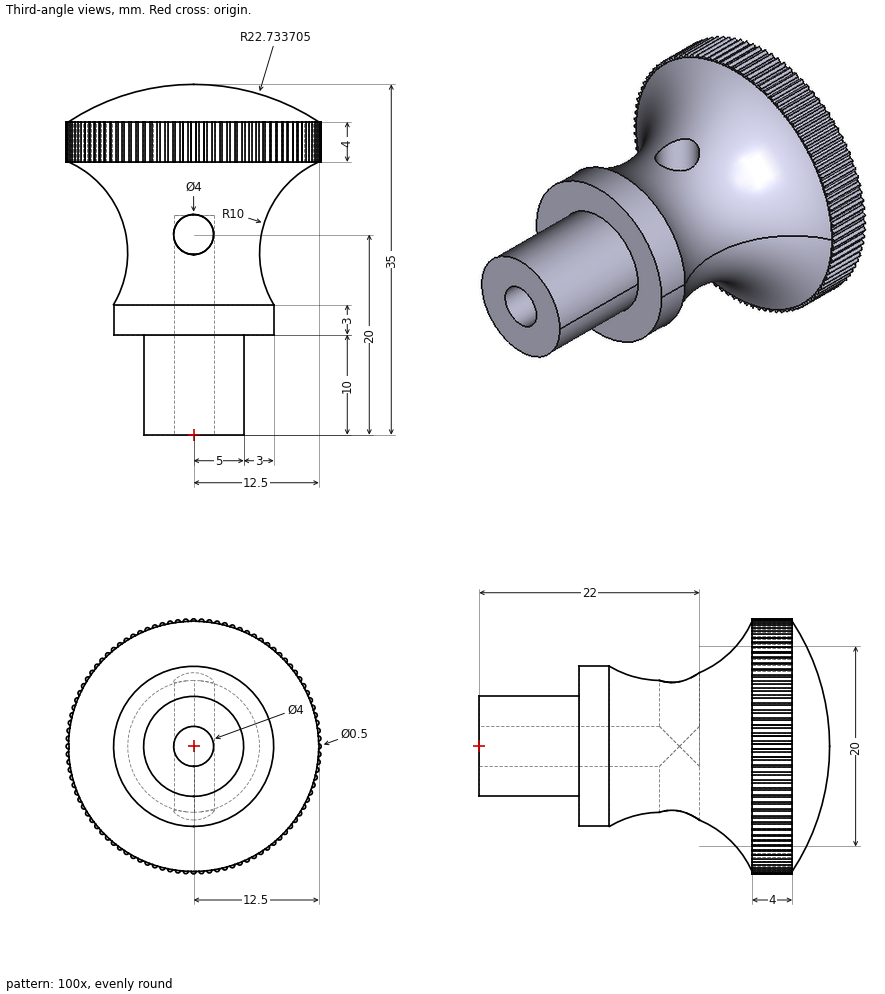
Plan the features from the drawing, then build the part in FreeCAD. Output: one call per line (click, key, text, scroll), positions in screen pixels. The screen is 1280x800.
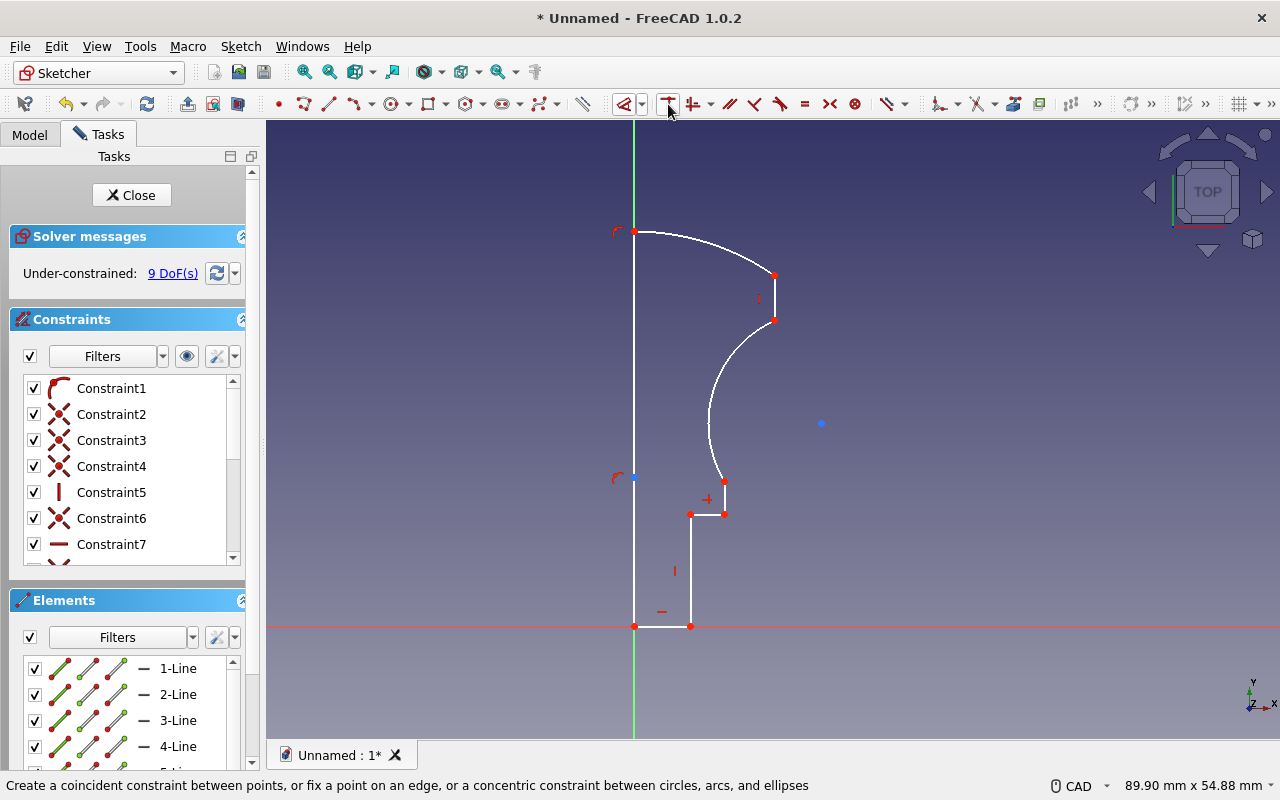
click(624, 104)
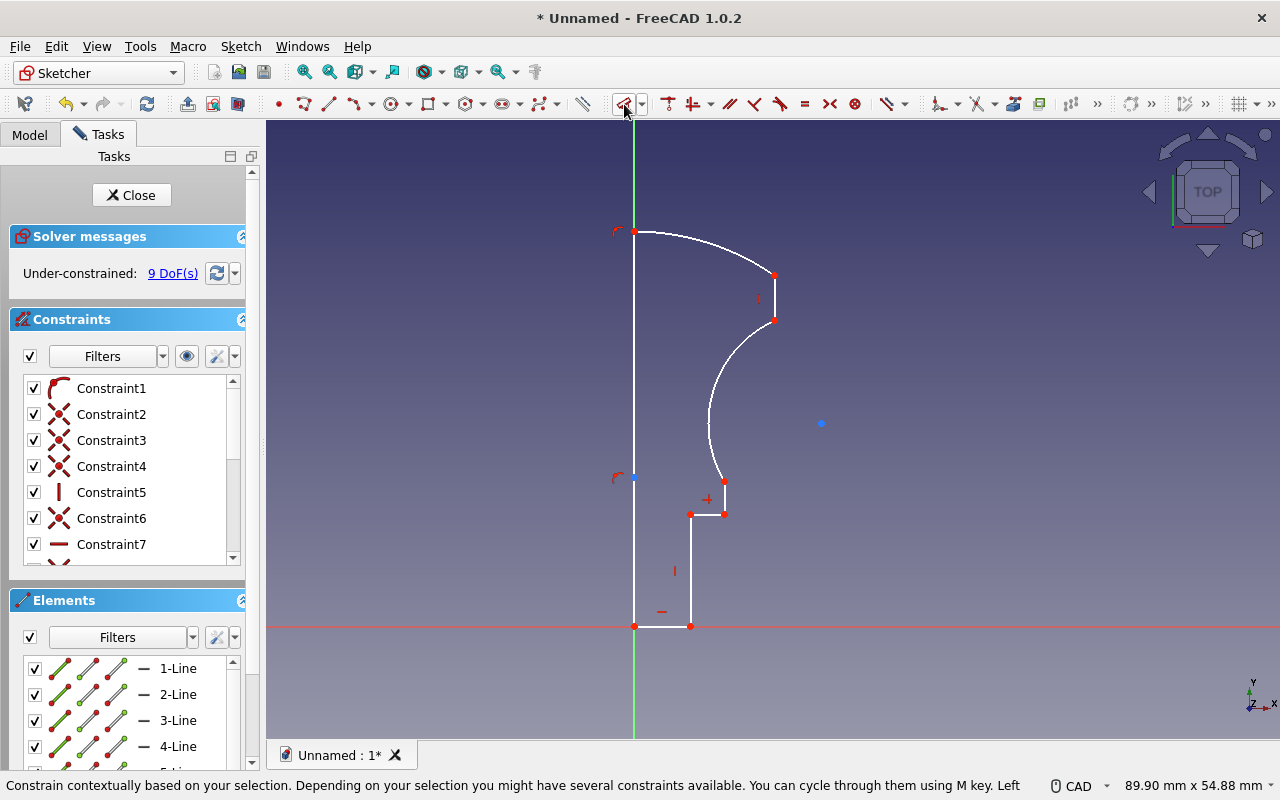
click(731, 356)
click(705, 337)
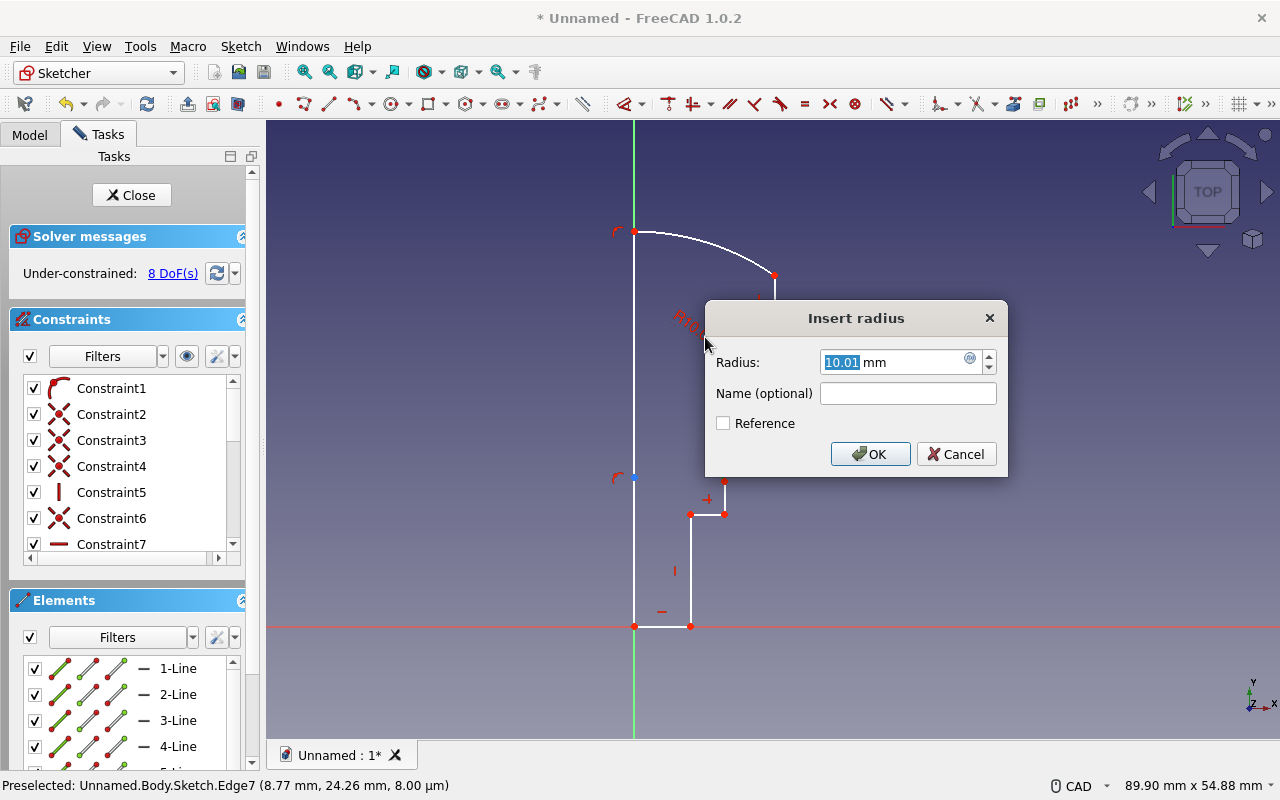
text(10)
key(Return)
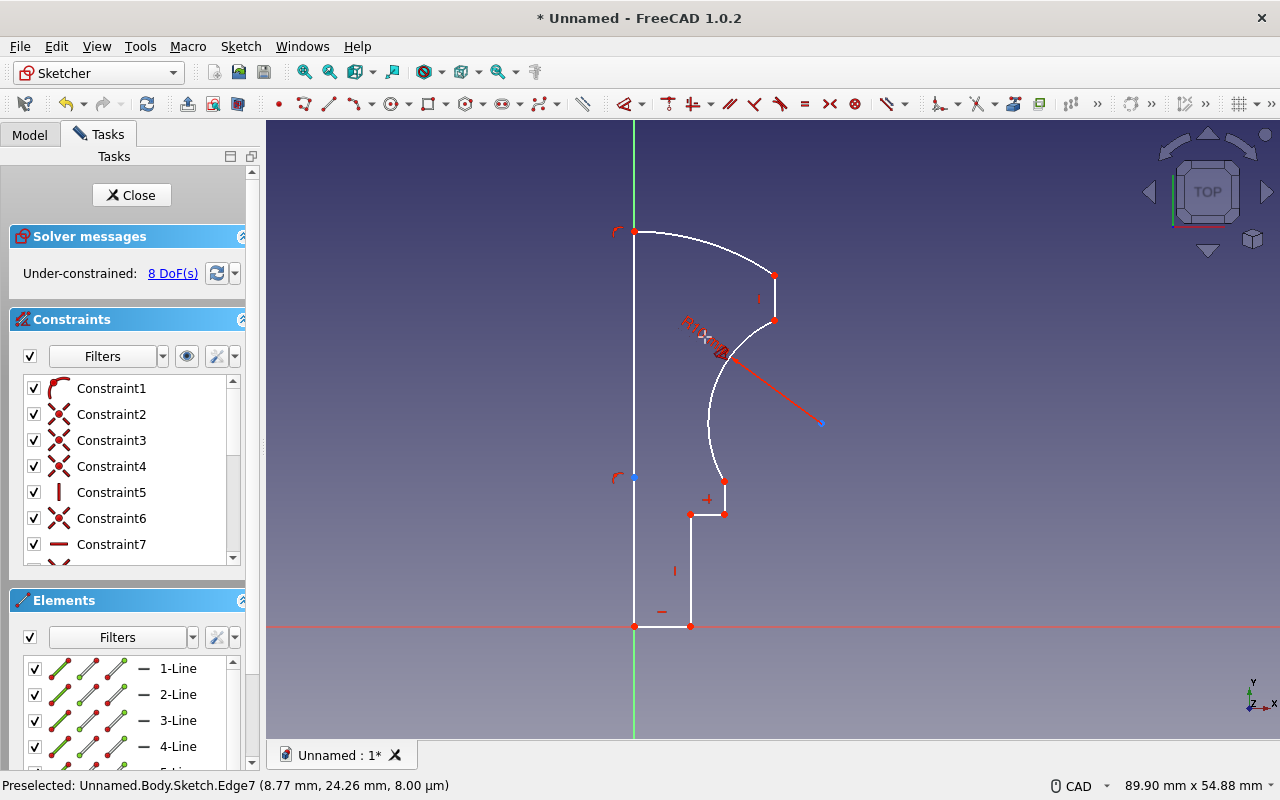
click(736, 254)
click(749, 225)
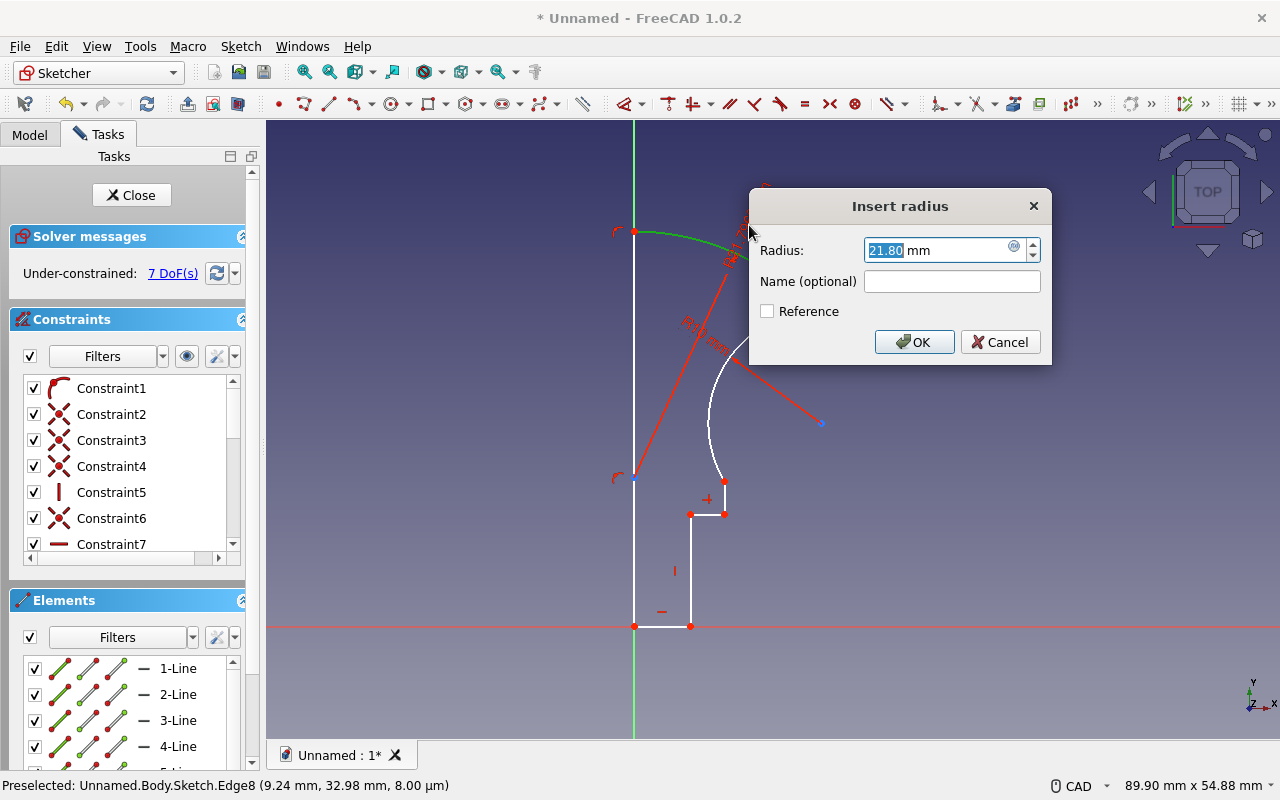
text(22.733705)
key(Return)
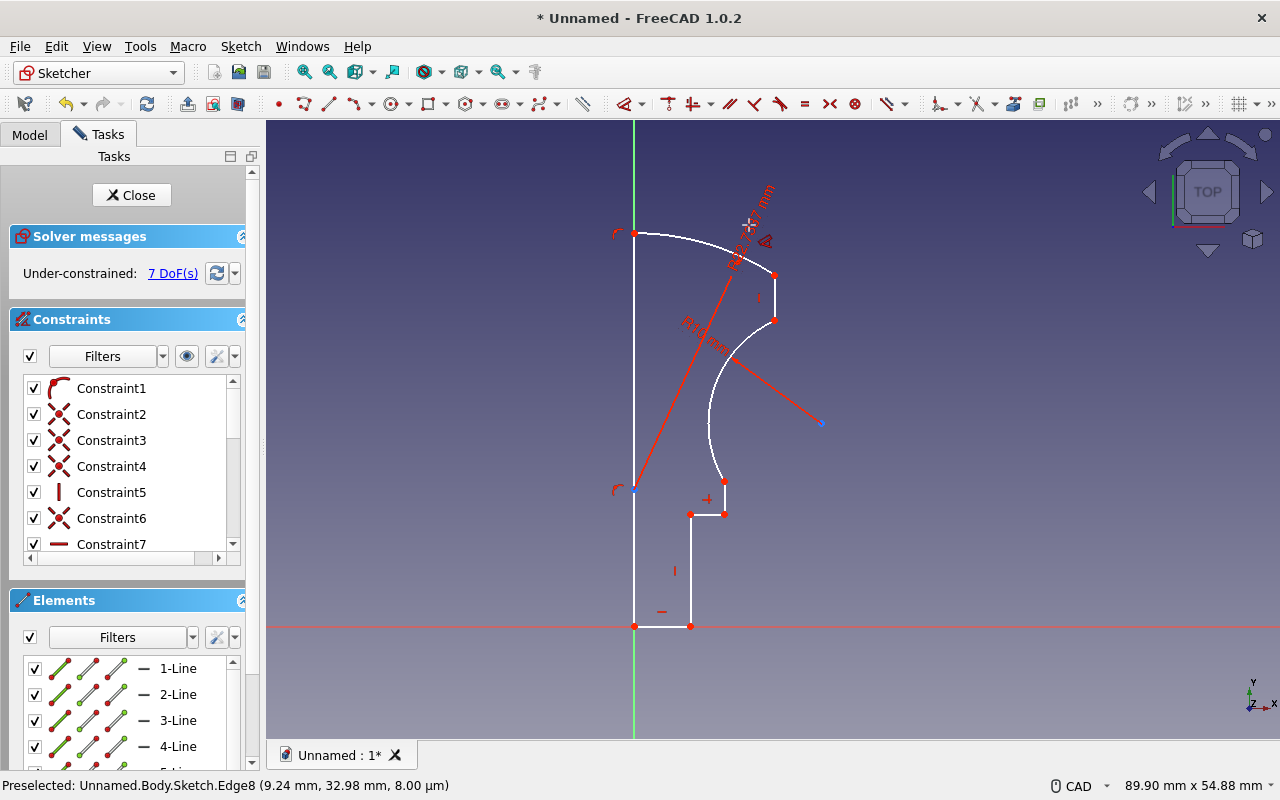
click(651, 627)
click(662, 661)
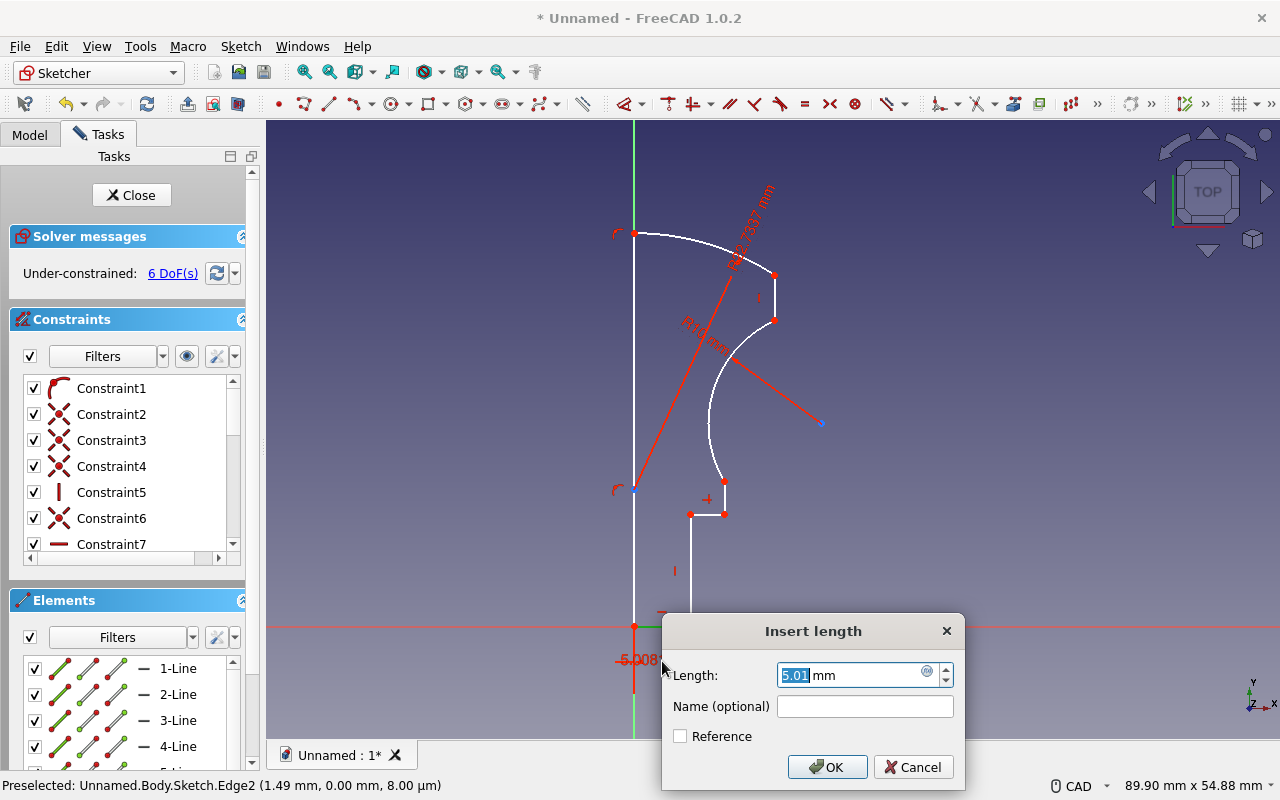
text(5)
key(Return)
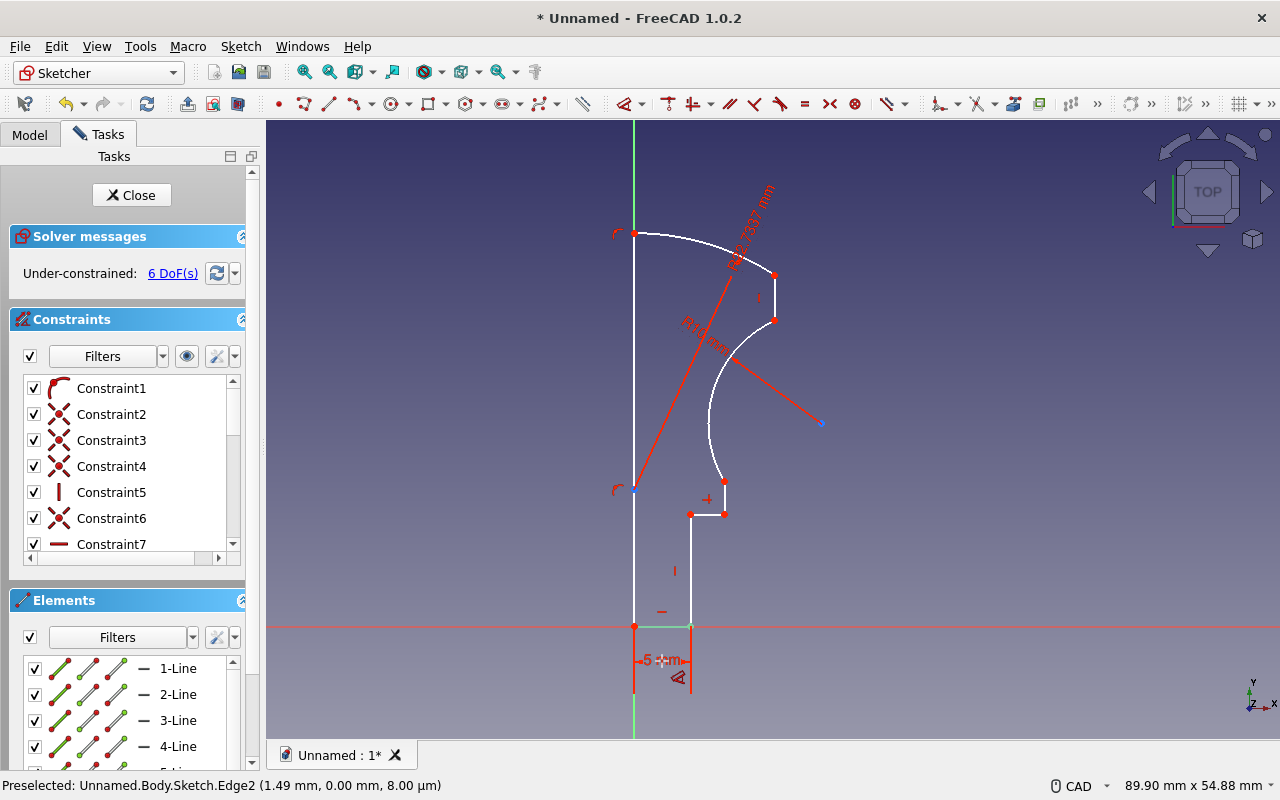
scroll(701, 515, up, 2)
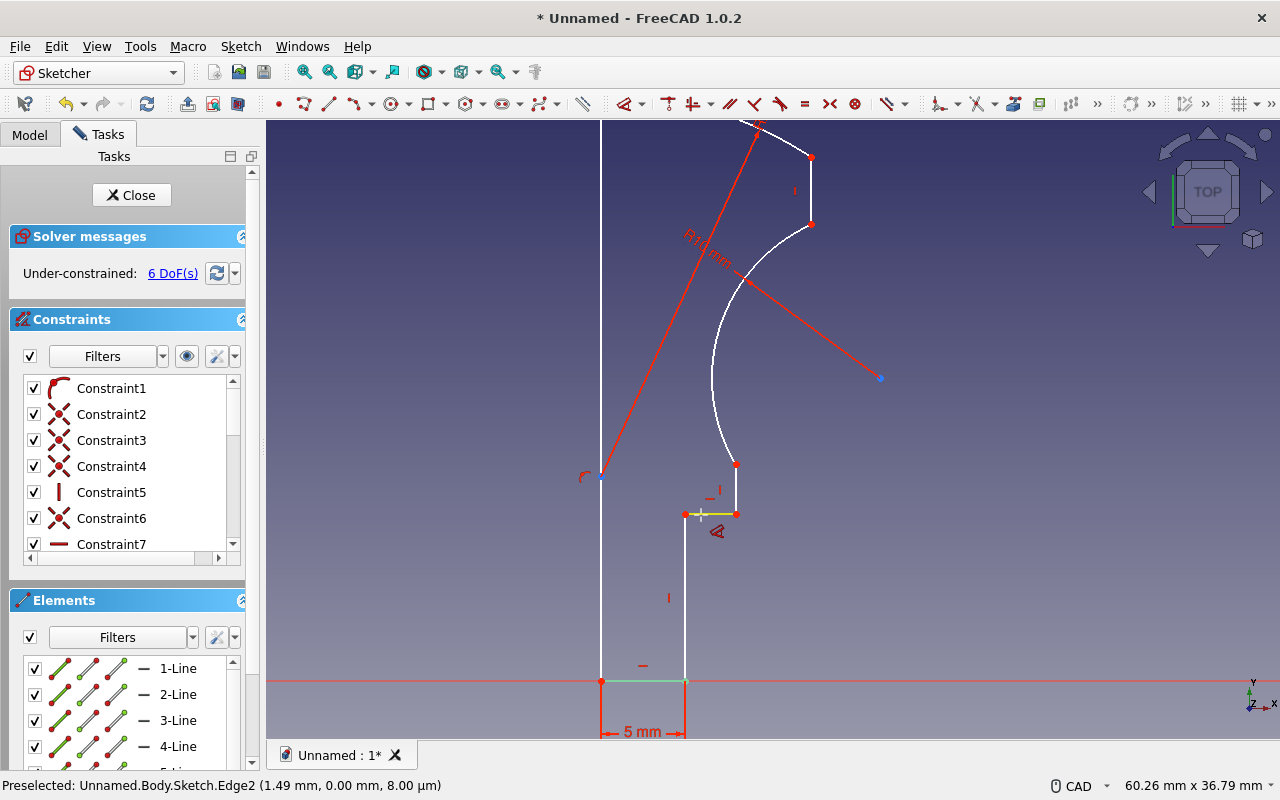
click(700, 514)
click(711, 548)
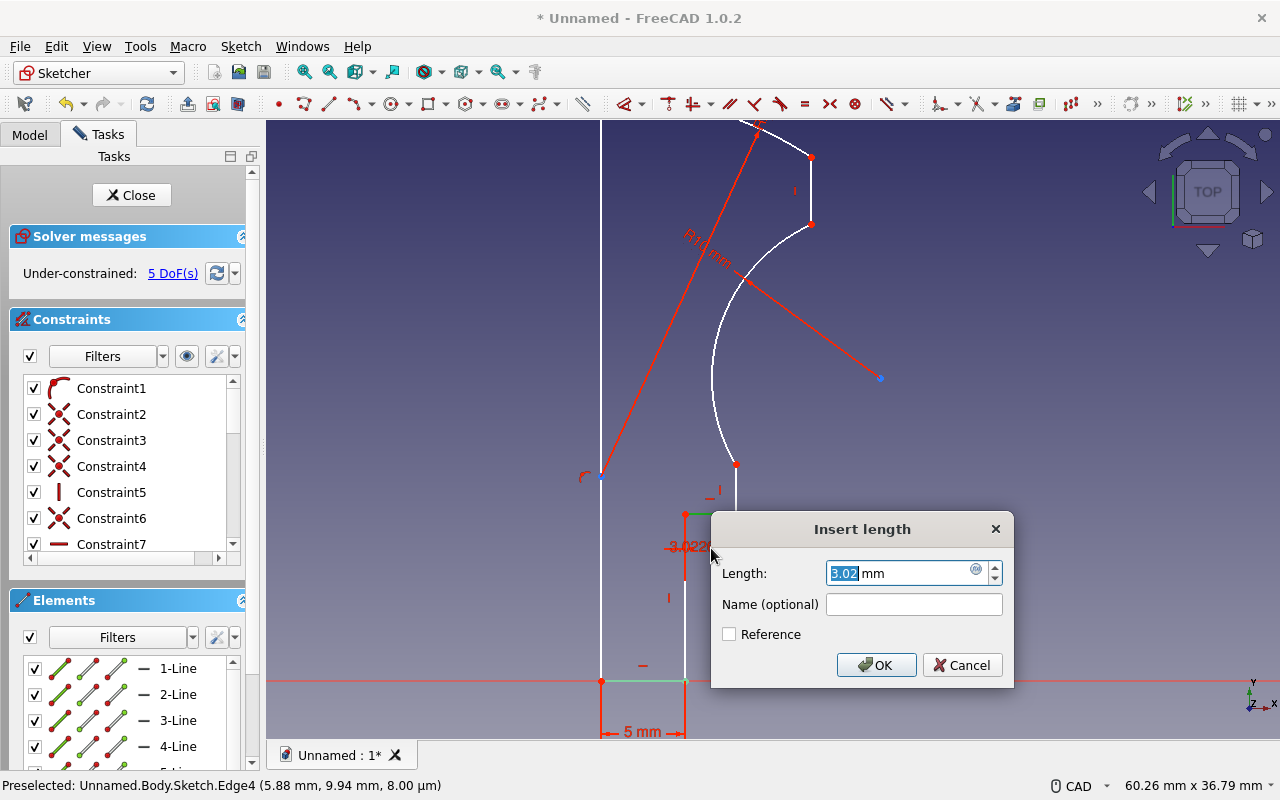
text(3)
key(Return)